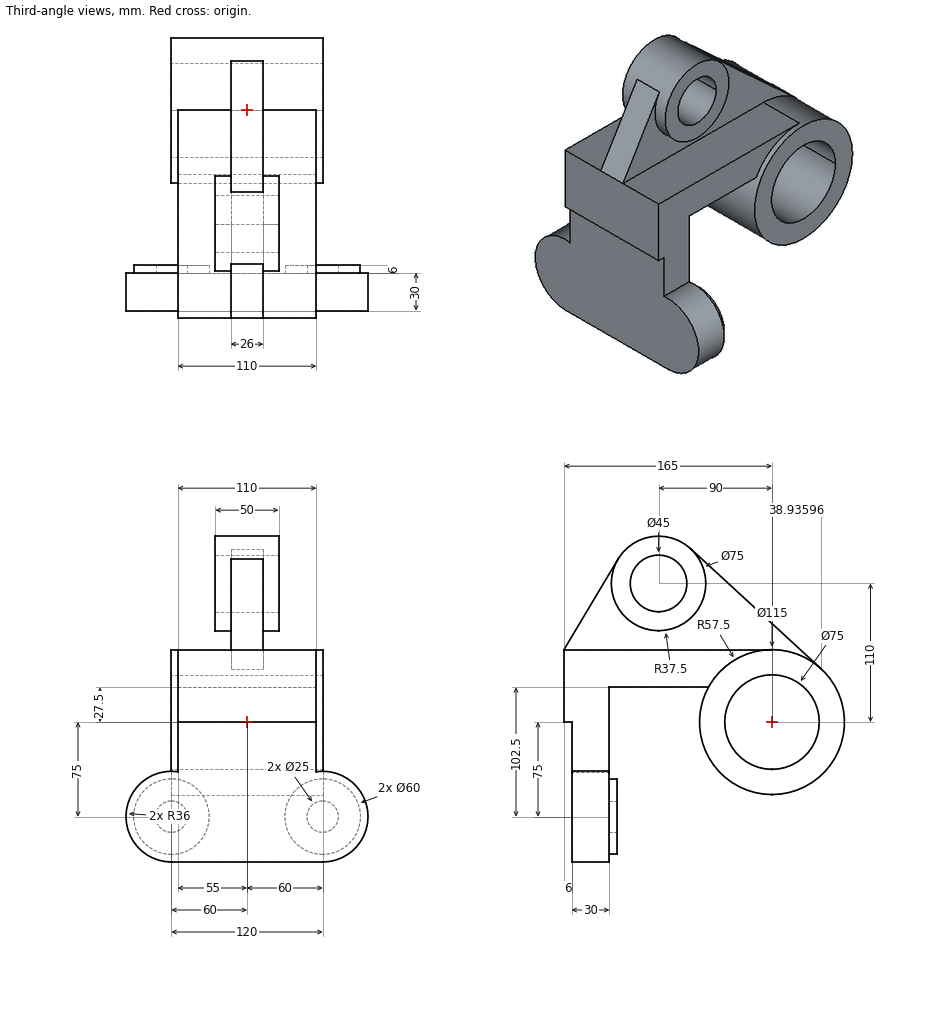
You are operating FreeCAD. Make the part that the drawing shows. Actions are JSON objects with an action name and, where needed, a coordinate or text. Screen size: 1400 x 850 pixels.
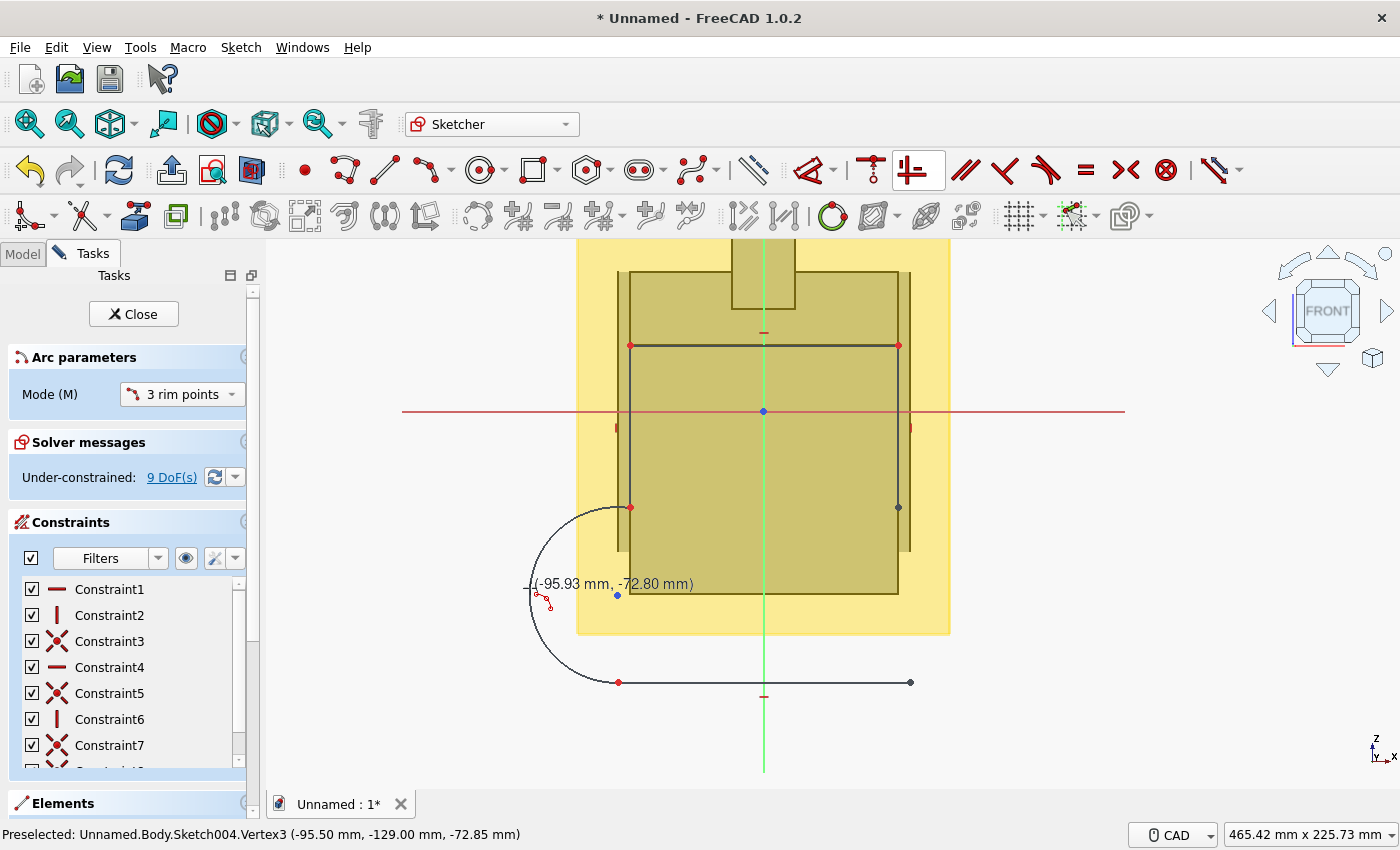
{"action": "left_click", "coordinate": [898, 508]}
{"action": "left_click", "coordinate": [910, 683]}
{"action": "left_click", "coordinate": [997, 588]}
{"action": "key", "text": "Escape"}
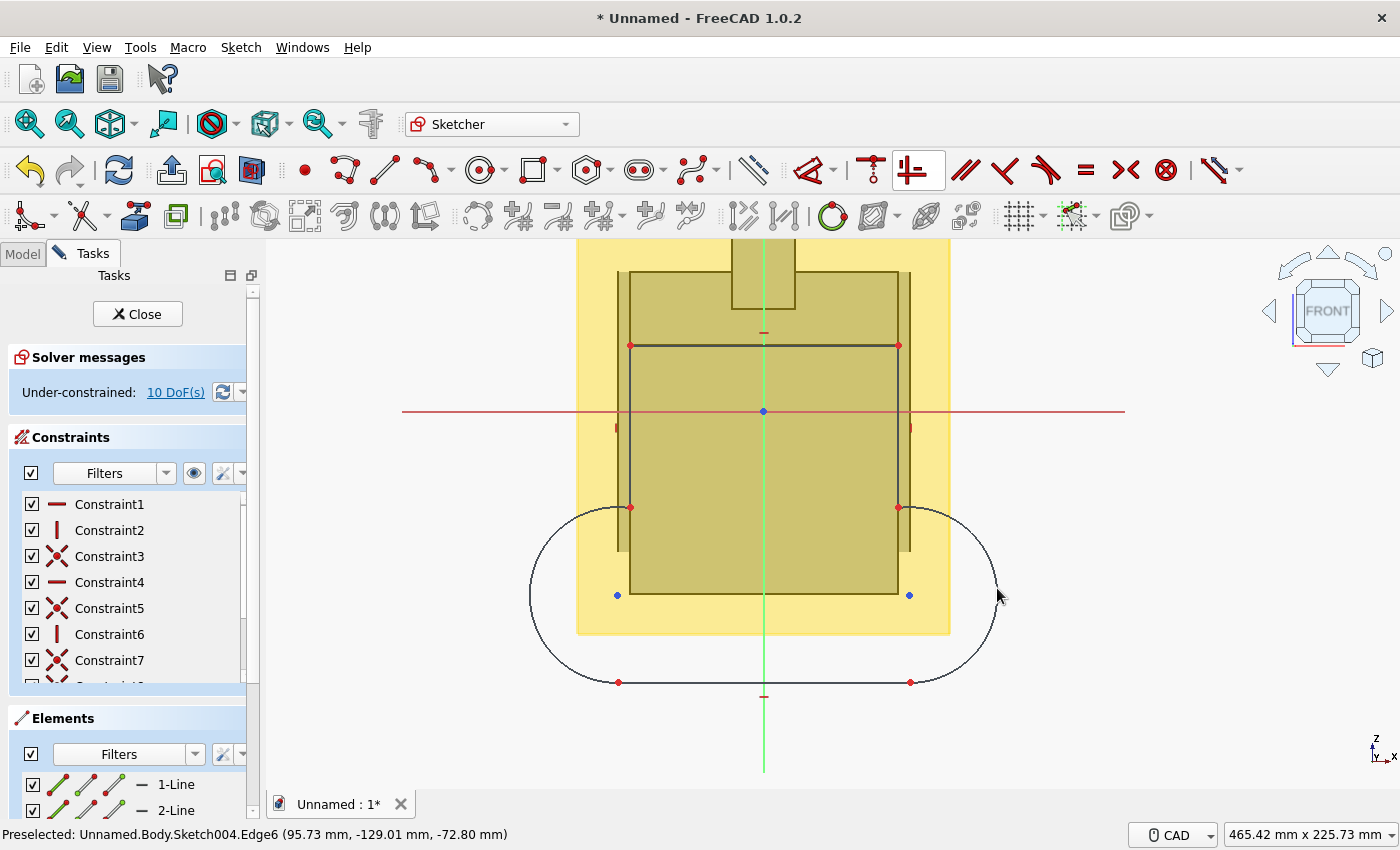
{"action": "left_click", "coordinate": [822, 683]}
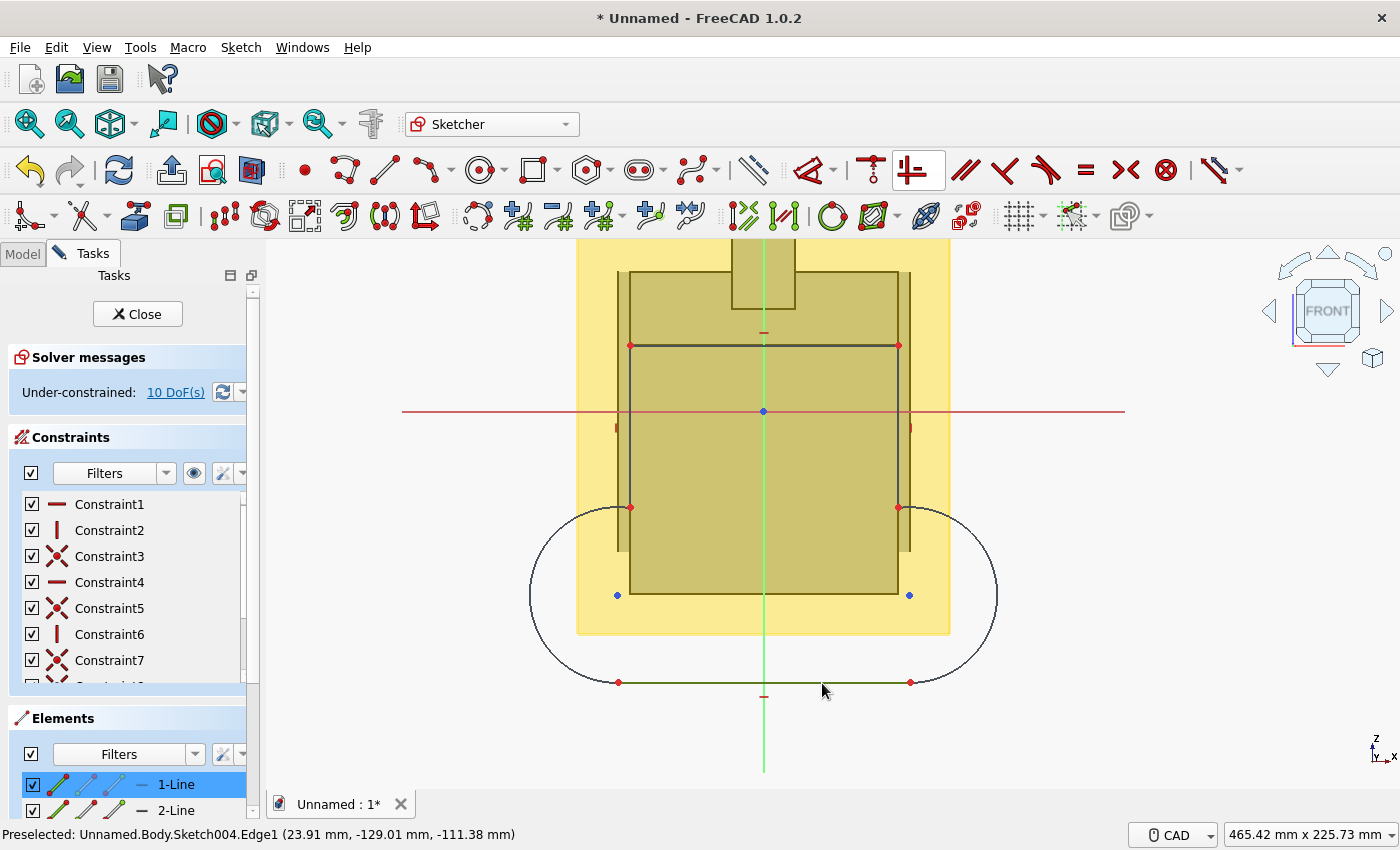
{"action": "left_click", "coordinate": [552, 537]}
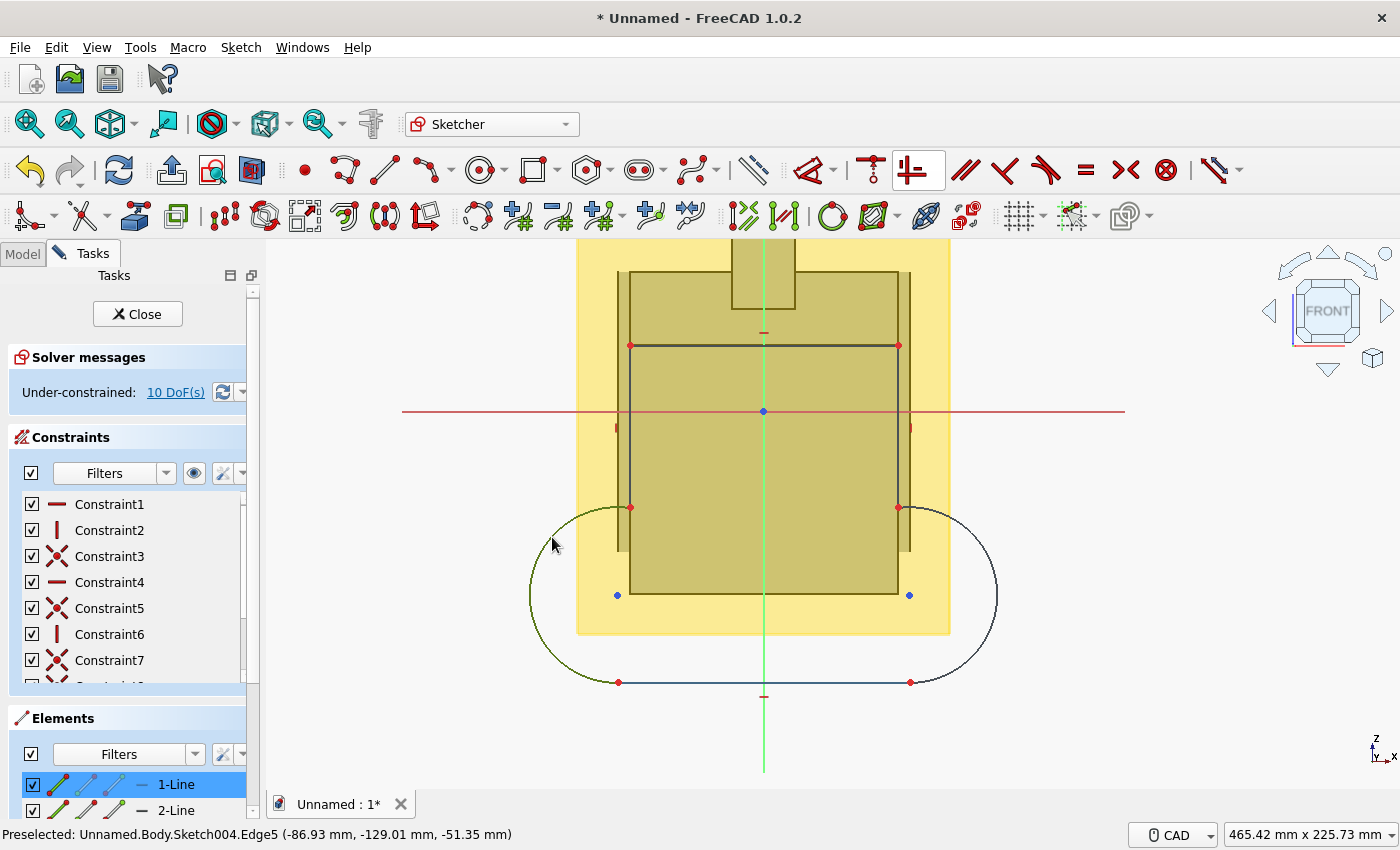
{"action": "left_click", "coordinate": [1046, 170]}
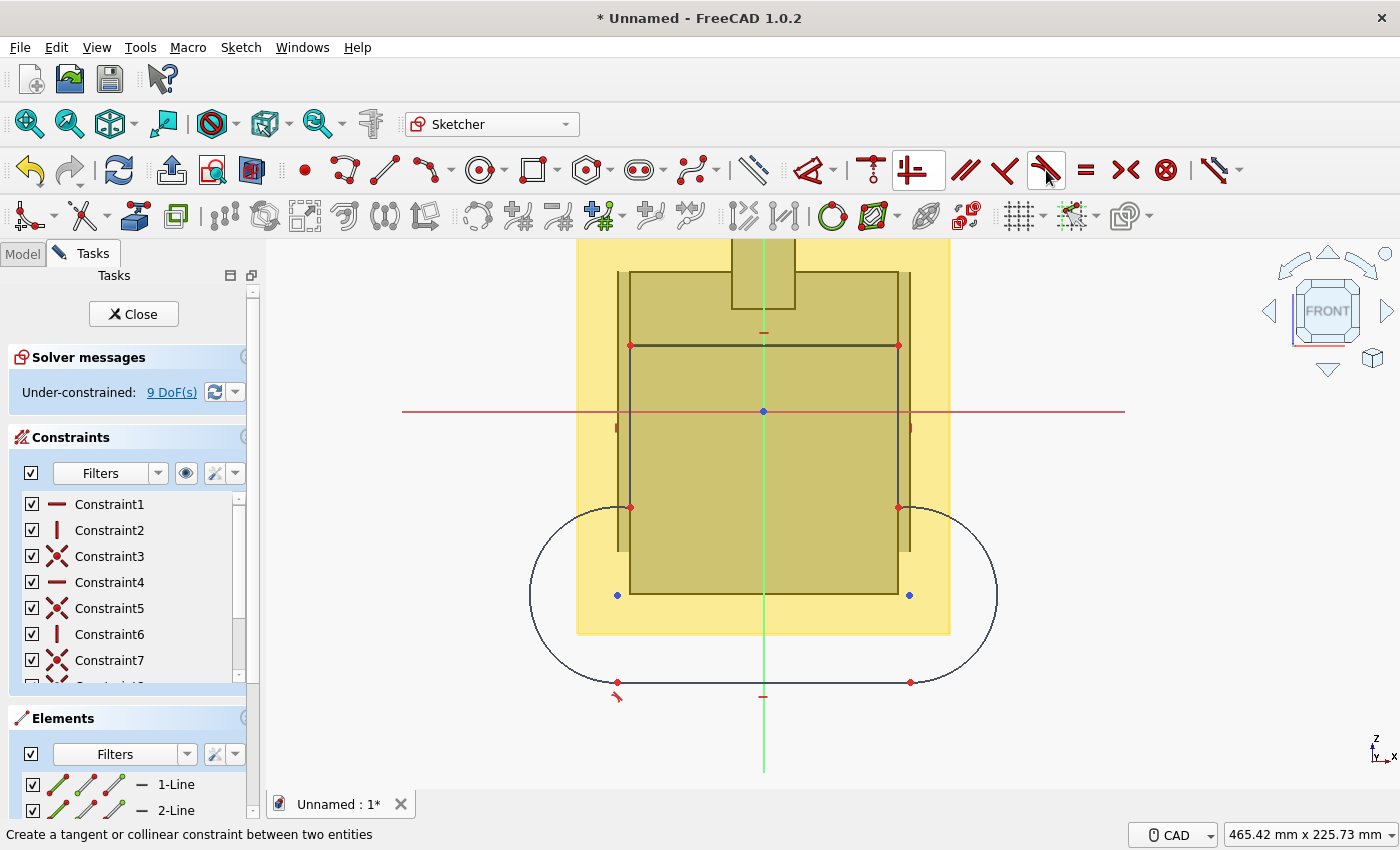
{"action": "left_click", "coordinate": [822, 683]}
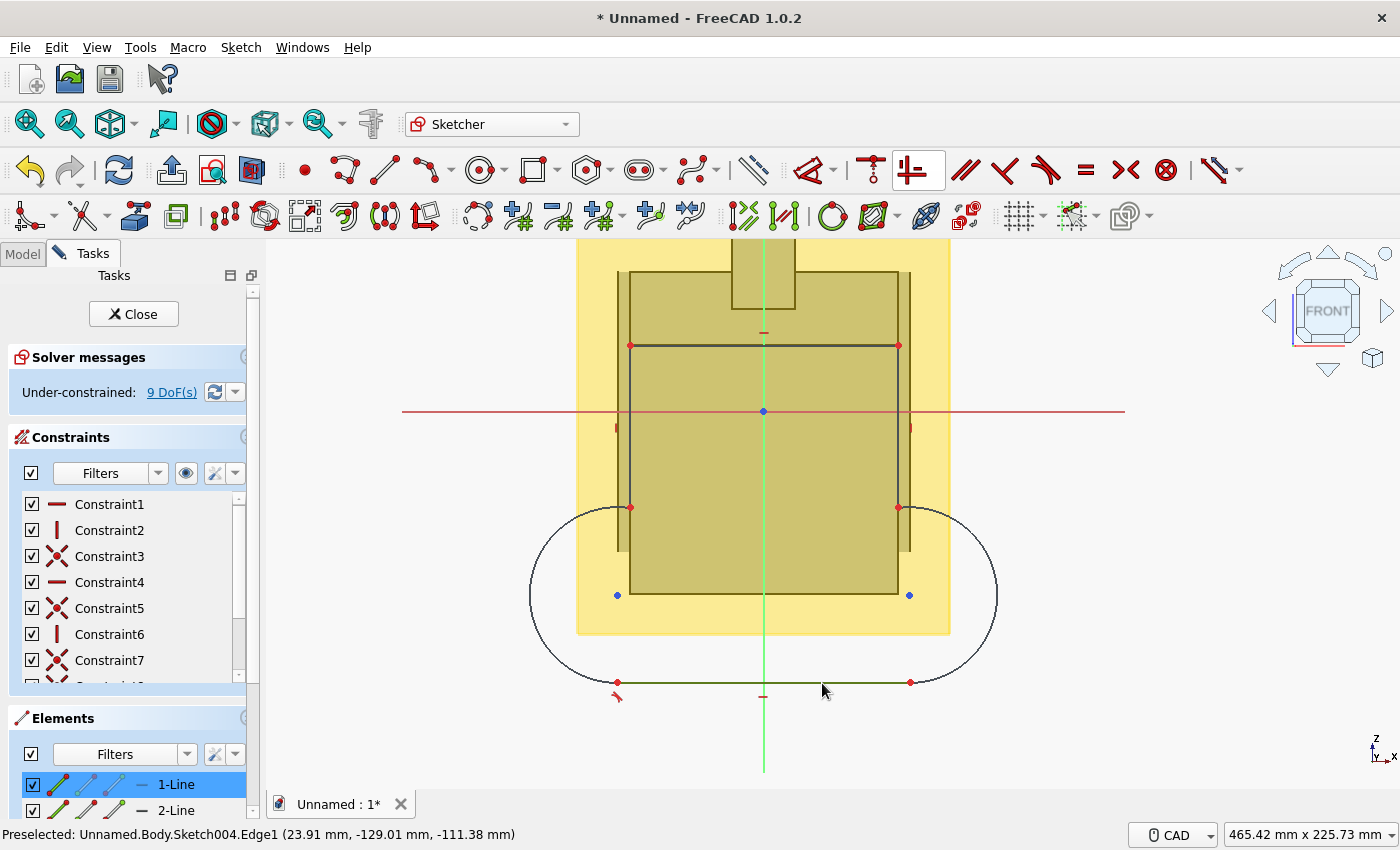
{"action": "left_click", "coordinate": [983, 644]}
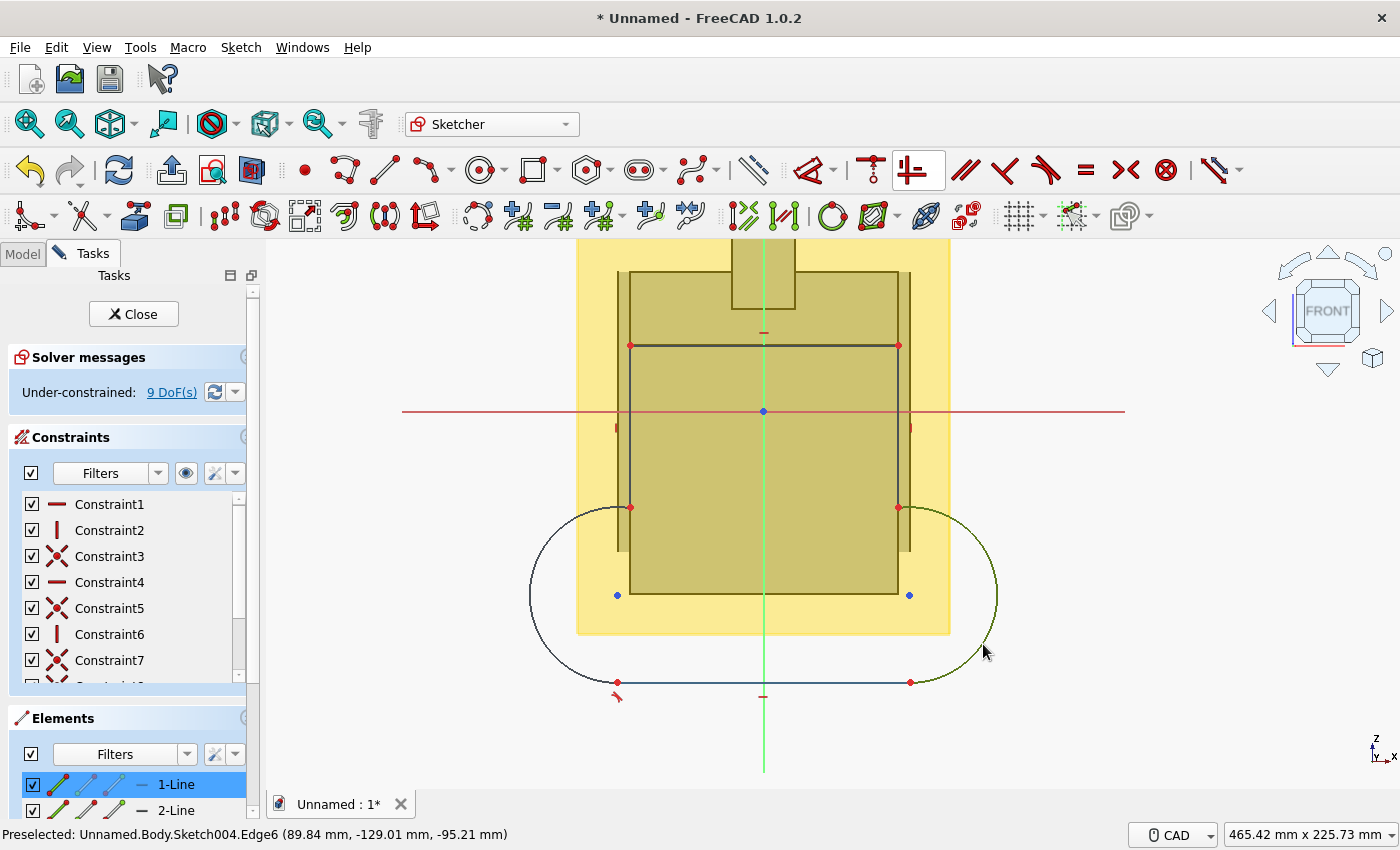
{"action": "left_click", "coordinate": [1046, 170]}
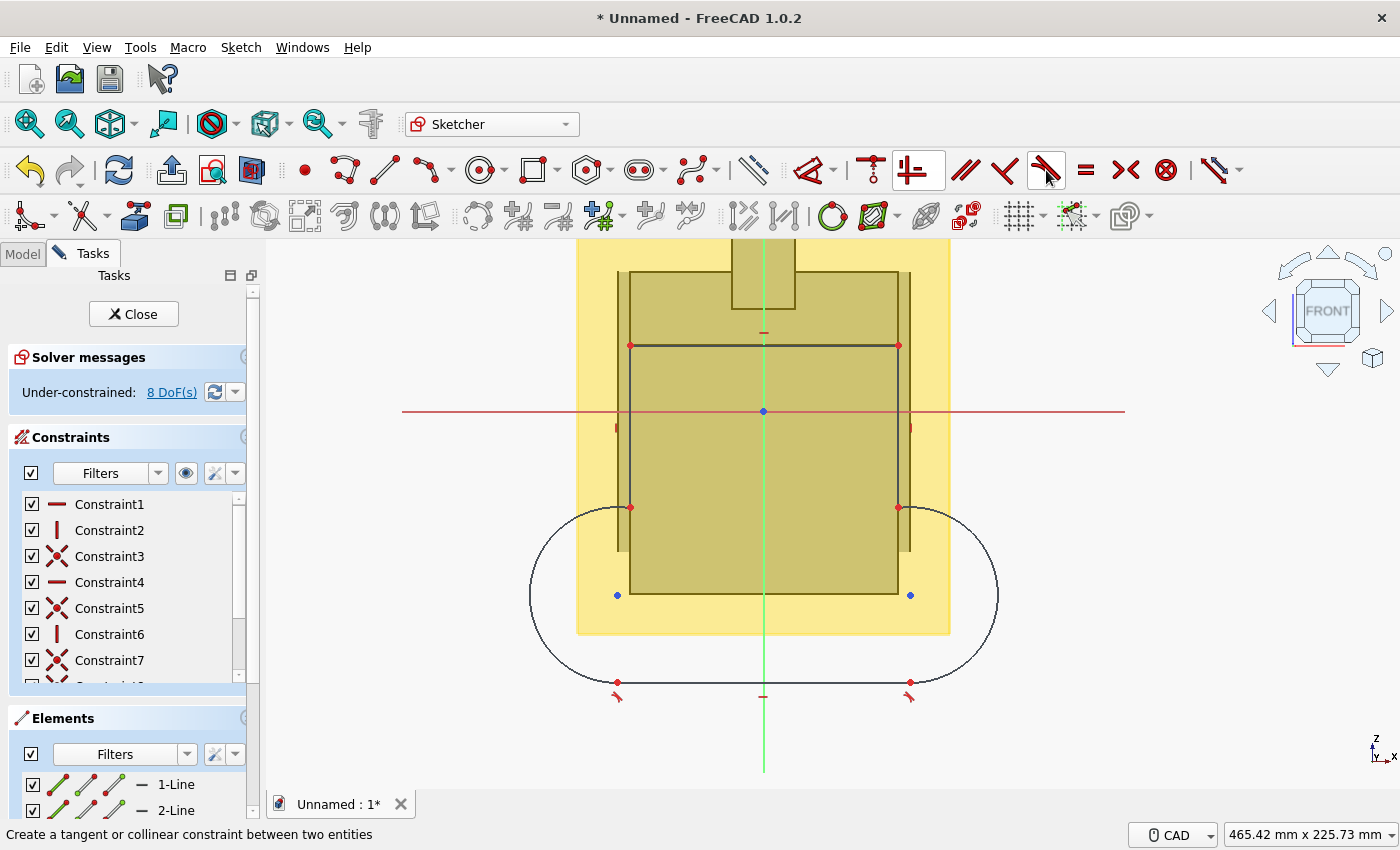
{"action": "left_click", "coordinate": [552, 537]}